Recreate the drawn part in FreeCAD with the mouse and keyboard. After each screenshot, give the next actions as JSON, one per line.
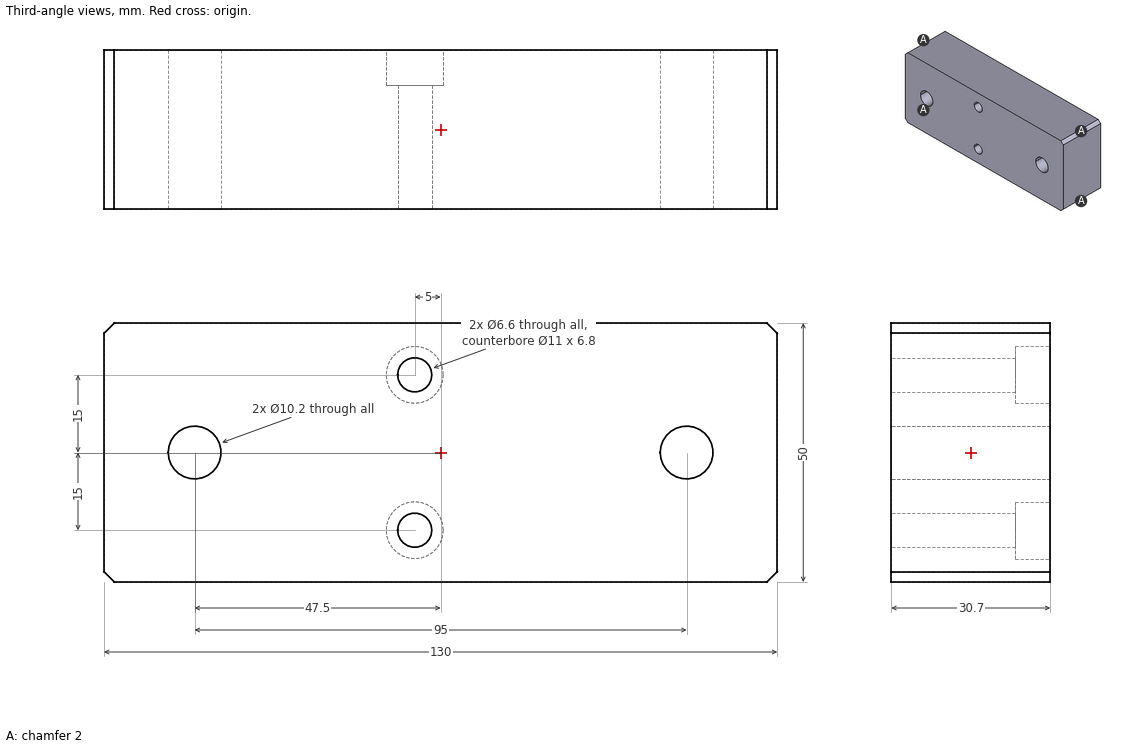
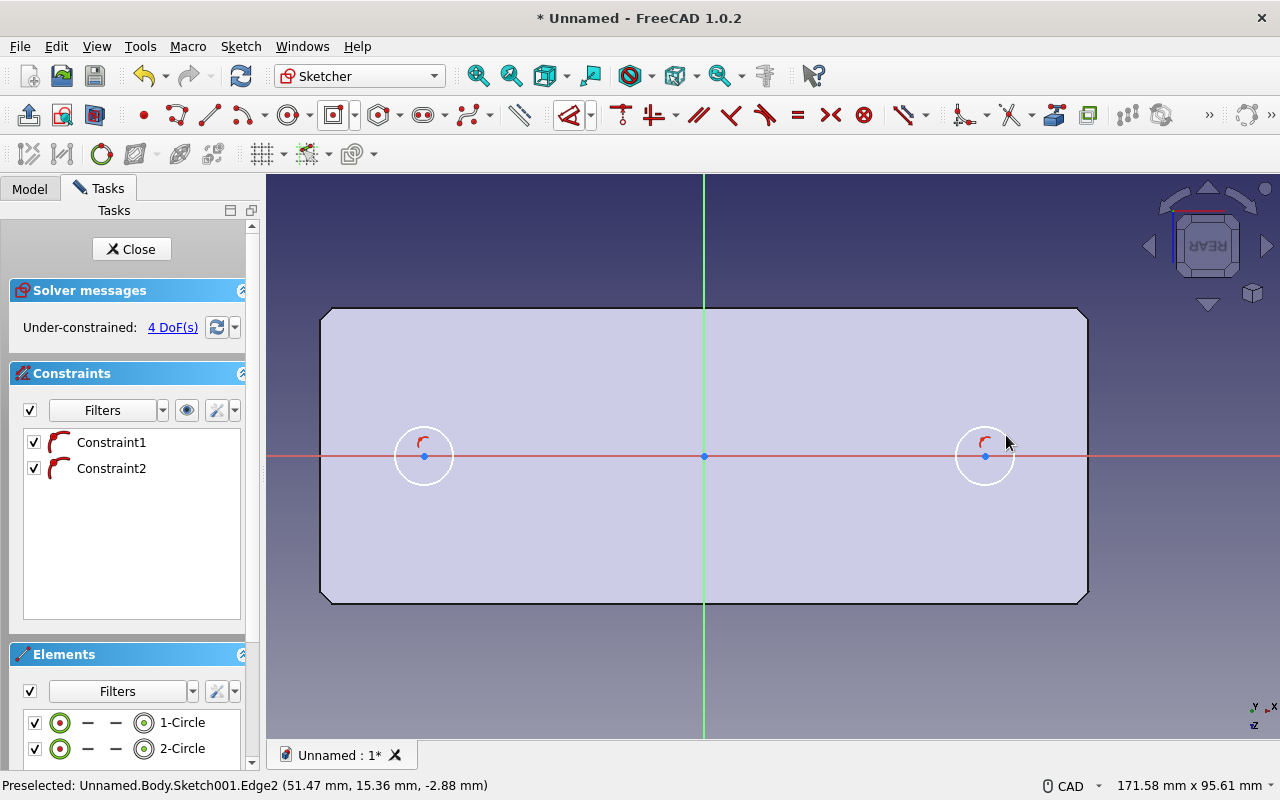
{"action": "left_click", "coordinate": [444, 435]}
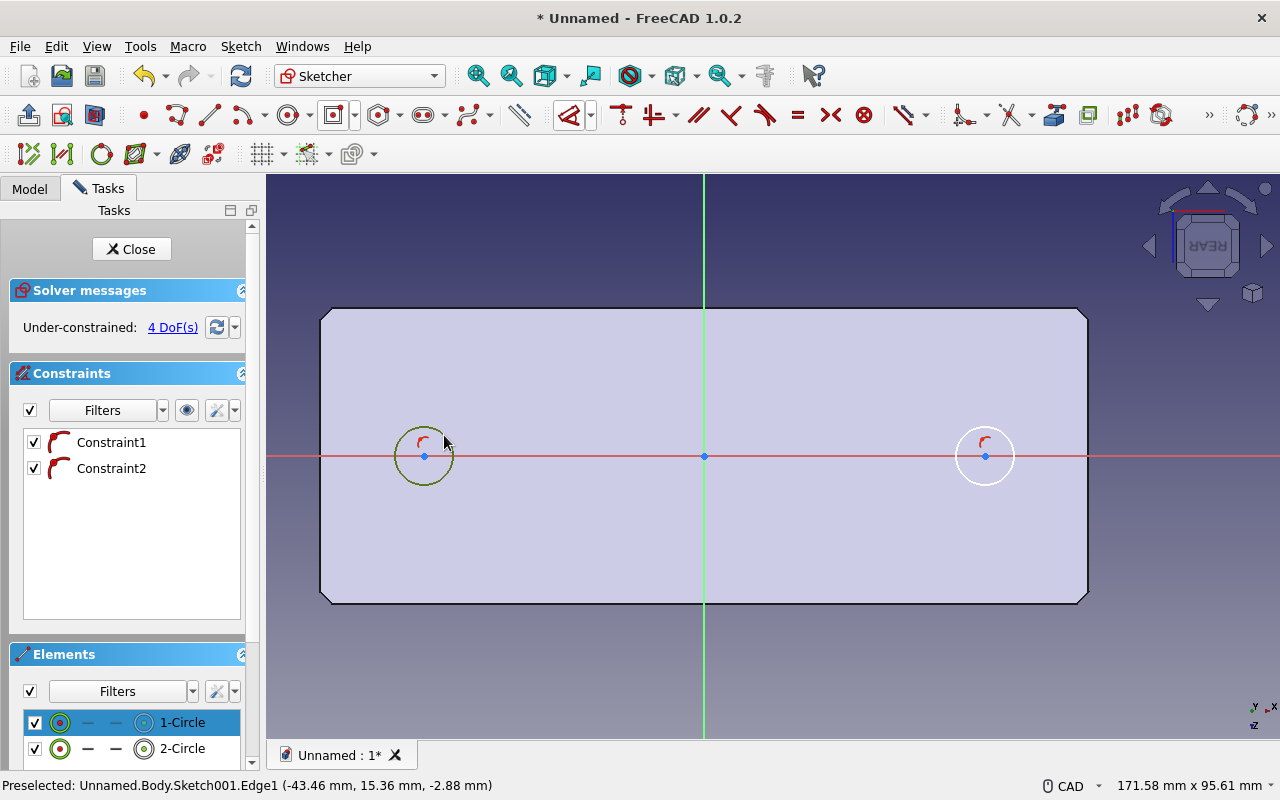
{"action": "left_click", "coordinate": [1005, 435]}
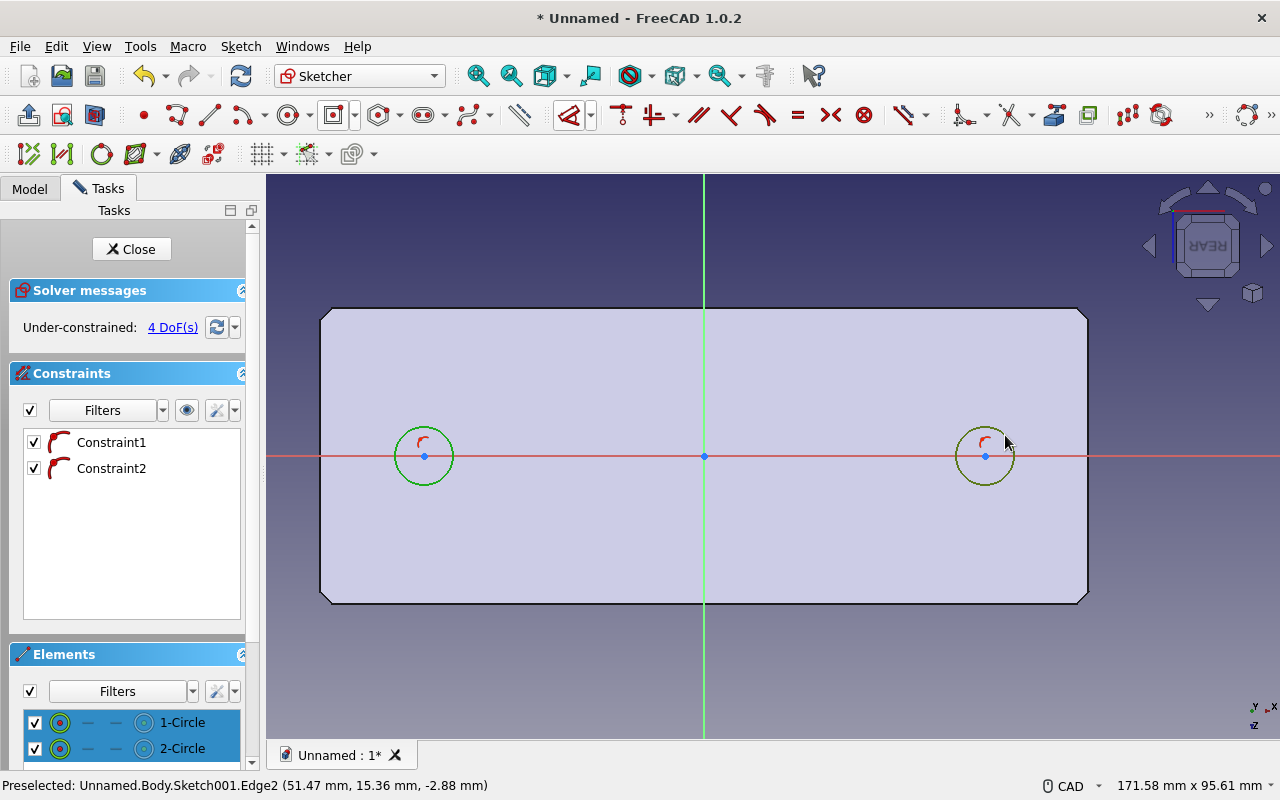
{"action": "left_click", "coordinate": [798, 116]}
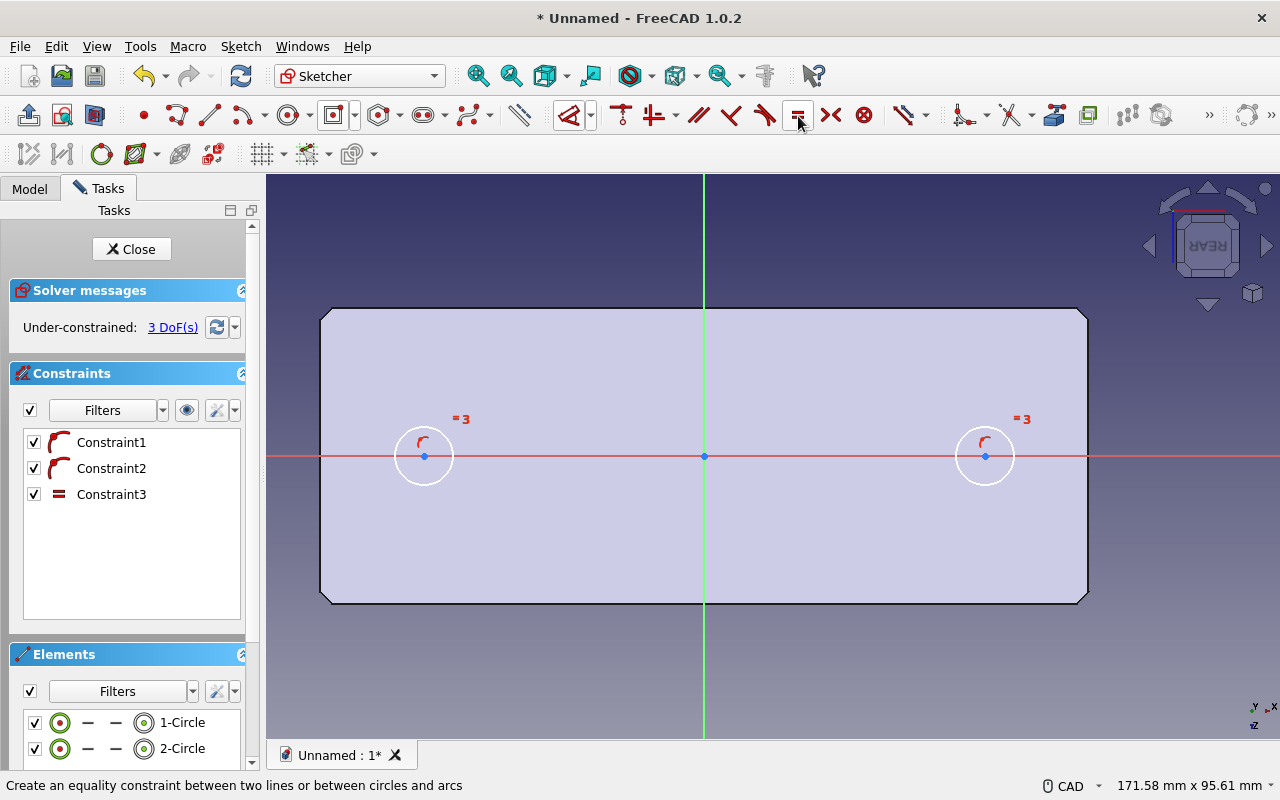
{"action": "left_click", "coordinate": [444, 435]}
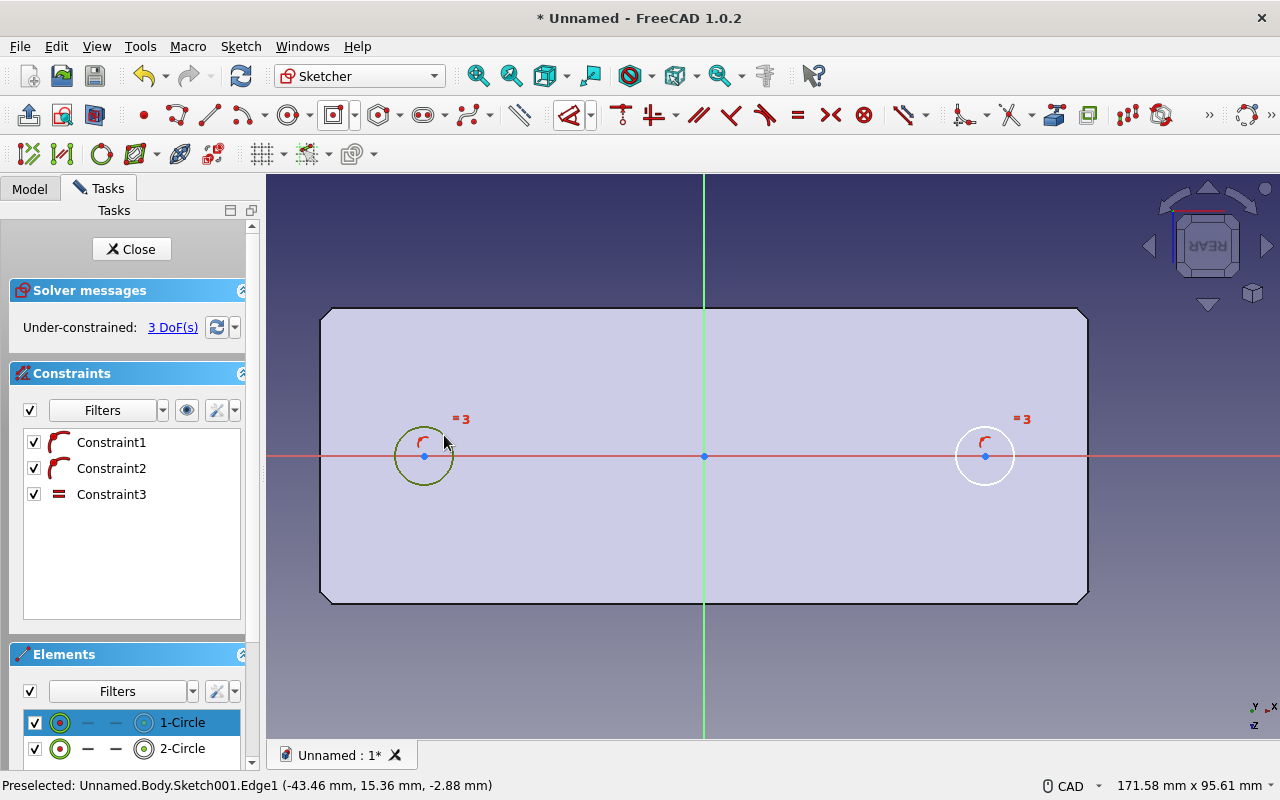
{"action": "left_click", "coordinate": [590, 116]}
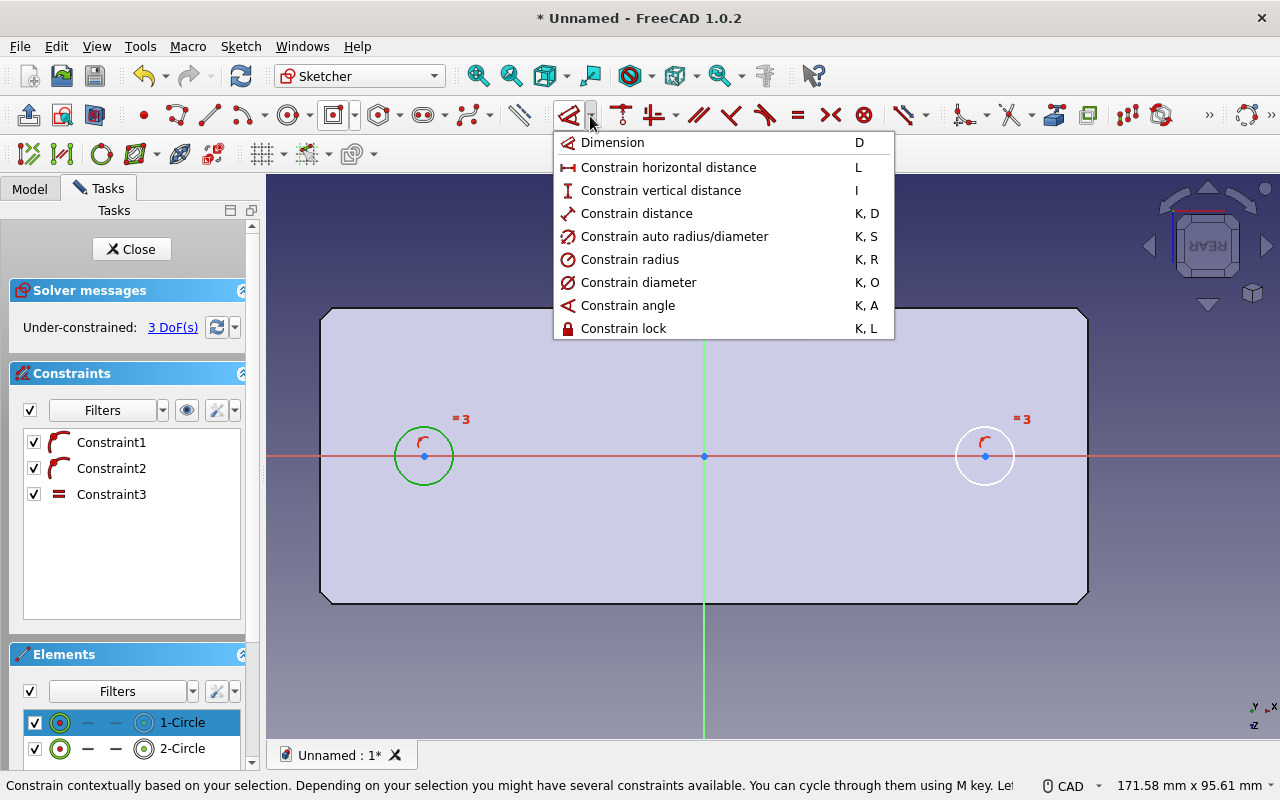
{"action": "left_click", "coordinate": [724, 282]}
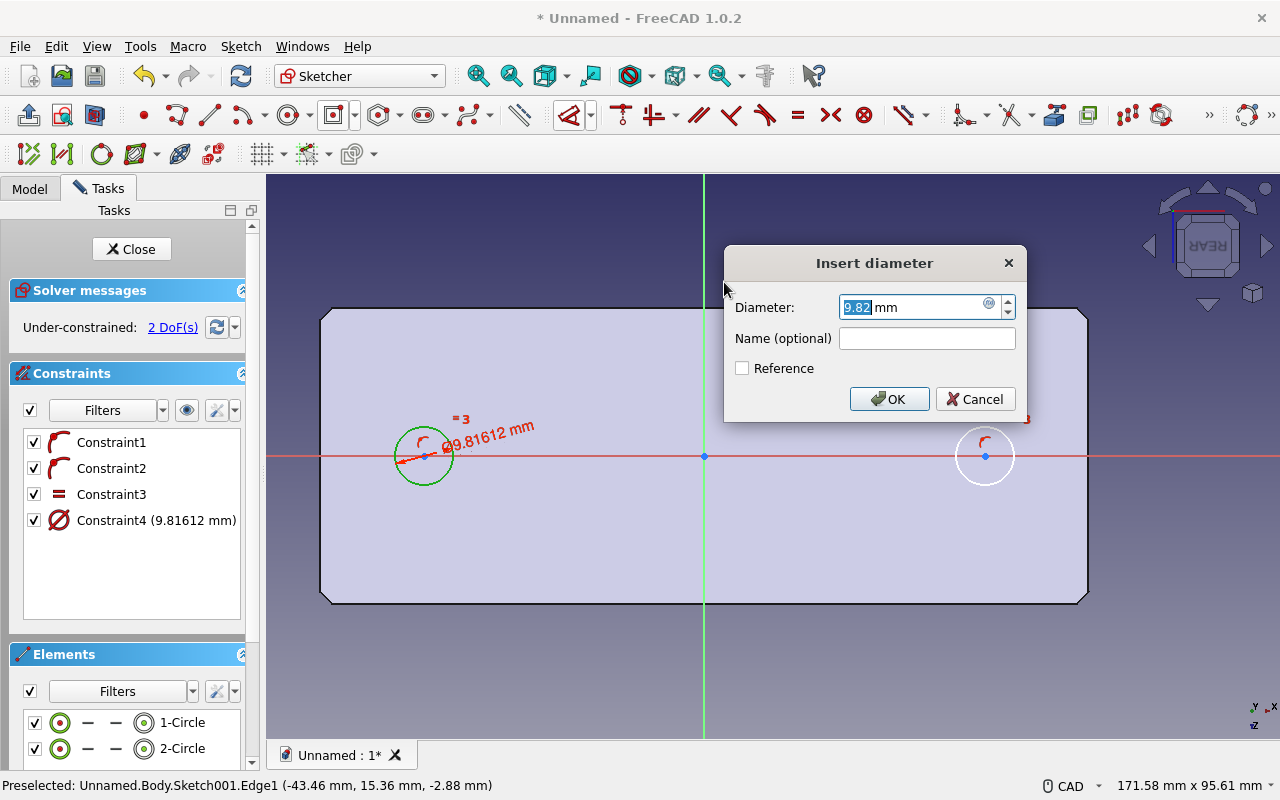
{"action": "type", "text": "10.2"}
{"action": "key", "text": "Return"}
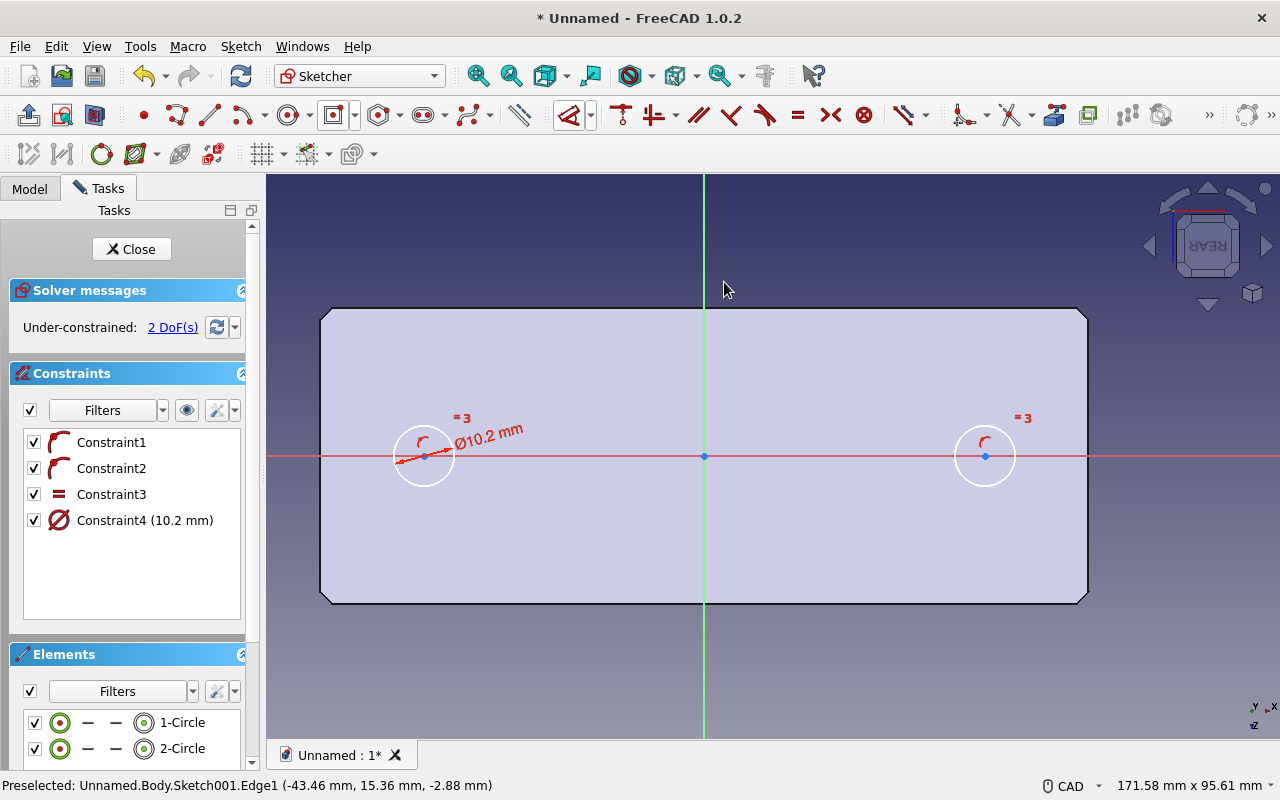
{"action": "left_click", "coordinate": [424, 456]}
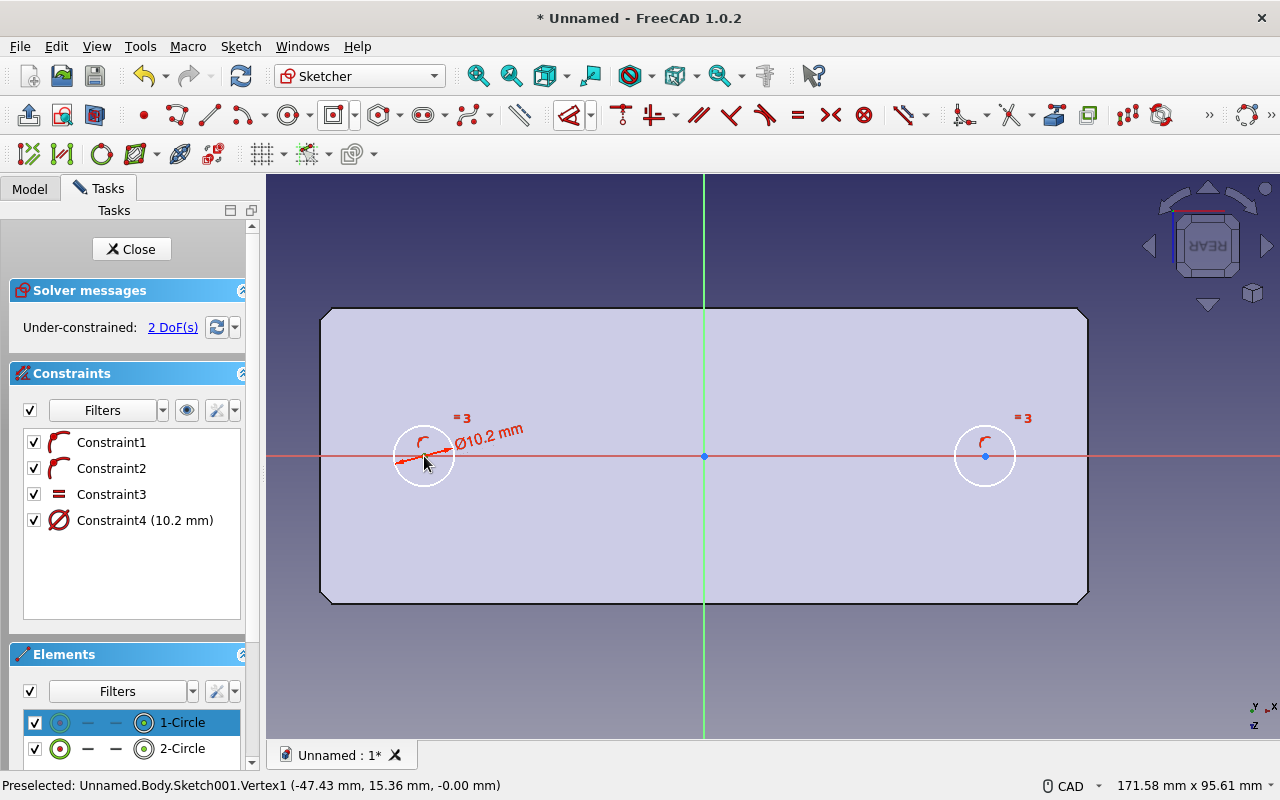
{"action": "left_click", "coordinate": [985, 456]}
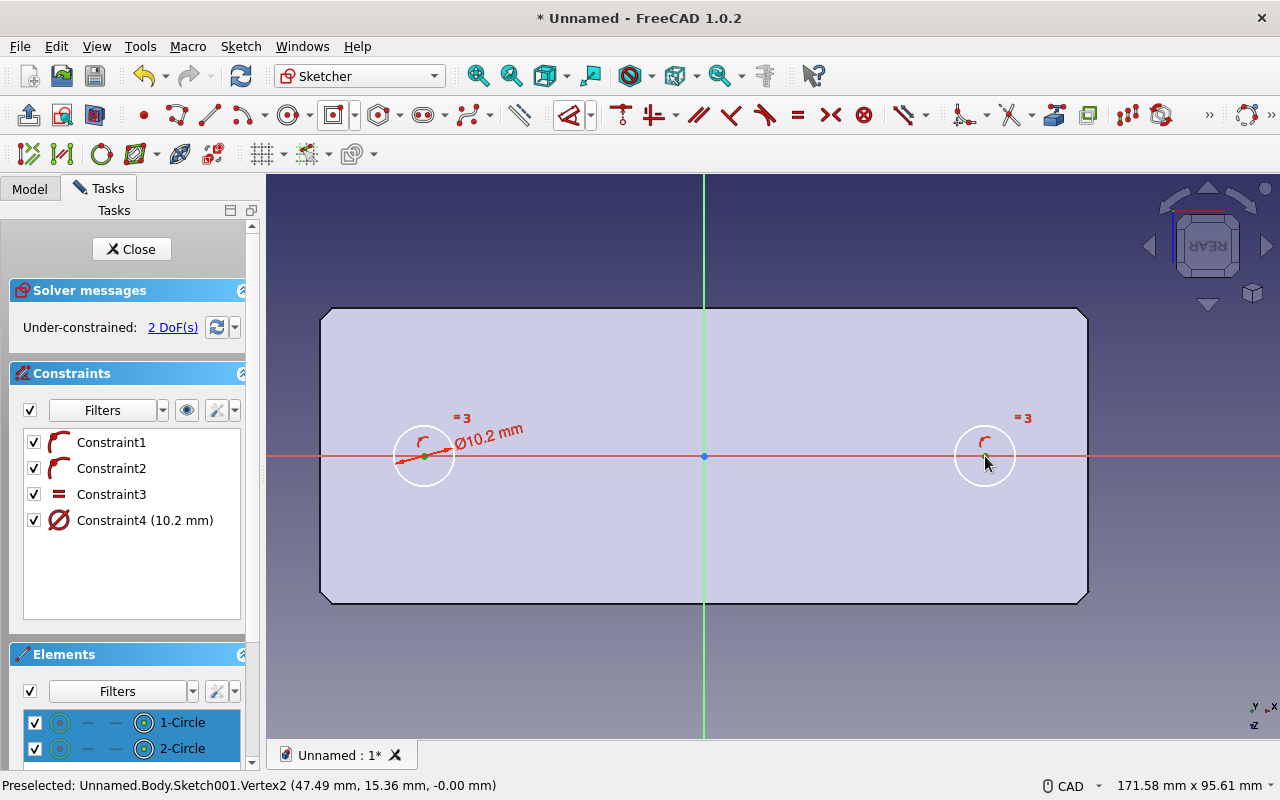
{"action": "key", "text": "l"}